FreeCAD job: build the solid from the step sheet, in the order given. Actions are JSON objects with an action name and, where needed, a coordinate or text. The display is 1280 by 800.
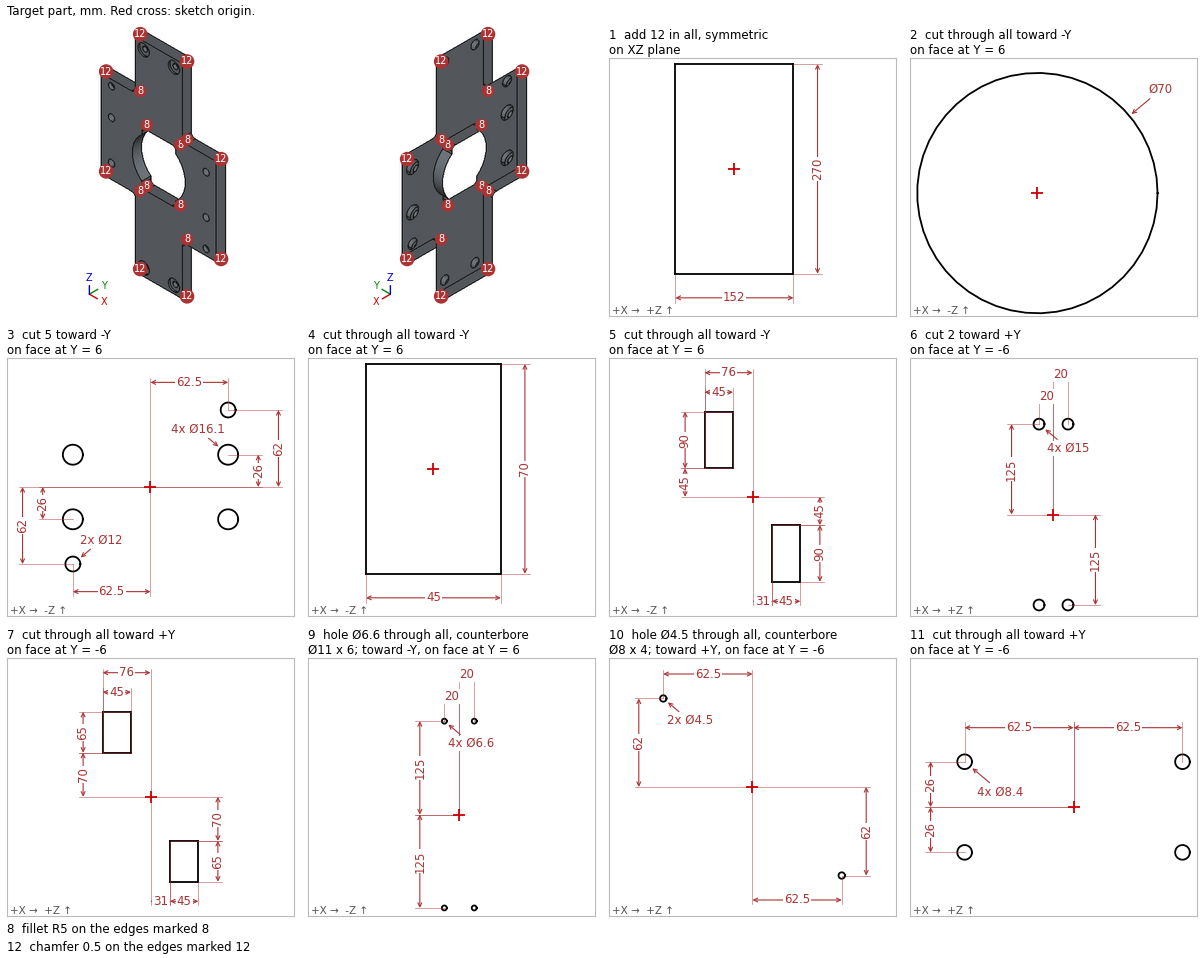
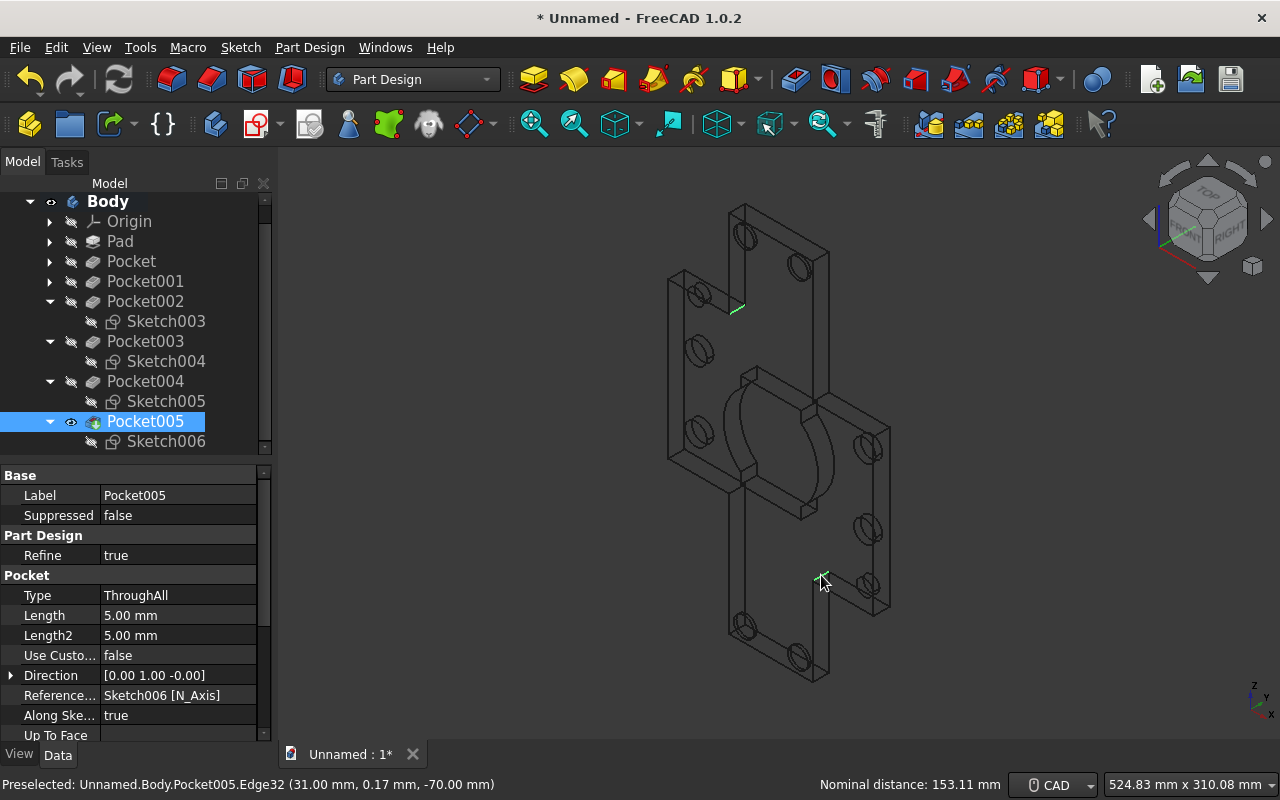
{"action": "left_click", "coordinate": [809, 514], "text": "ctrl"}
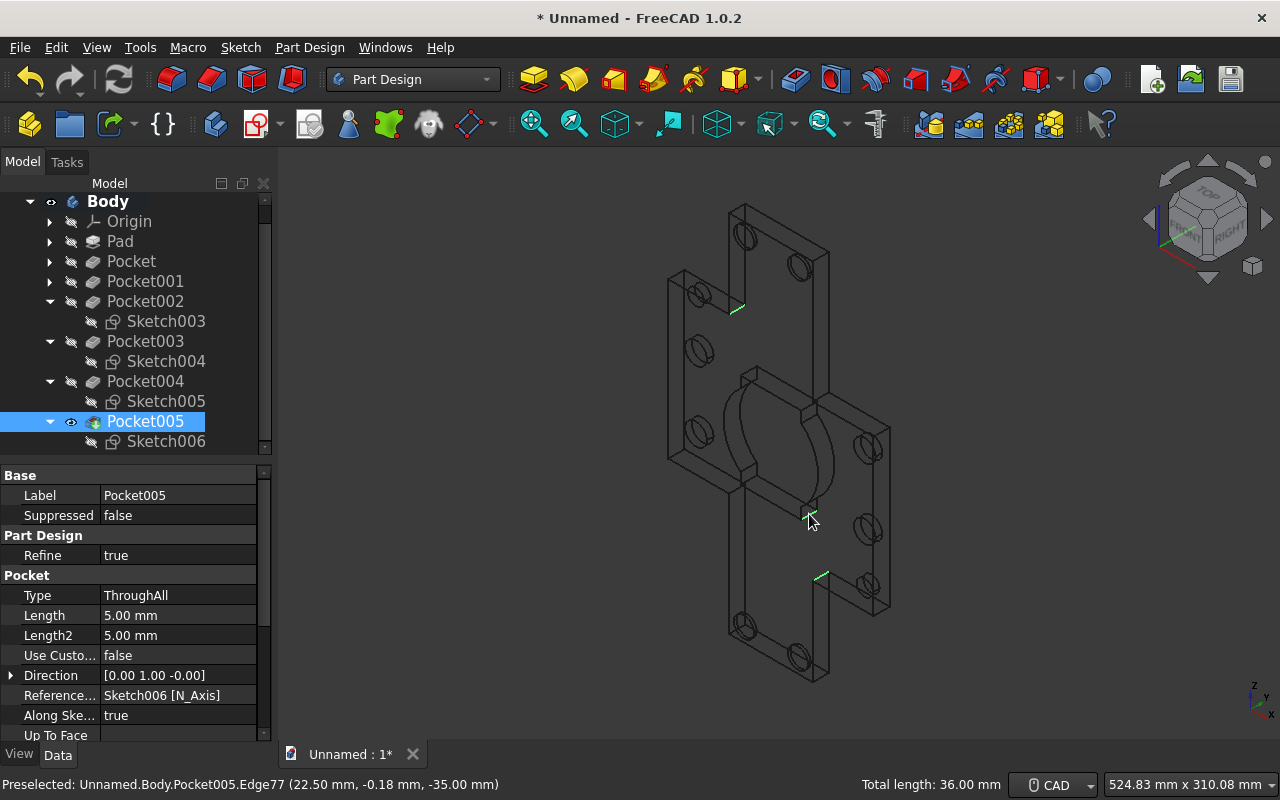
{"action": "left_click", "coordinate": [808, 406], "text": "ctrl"}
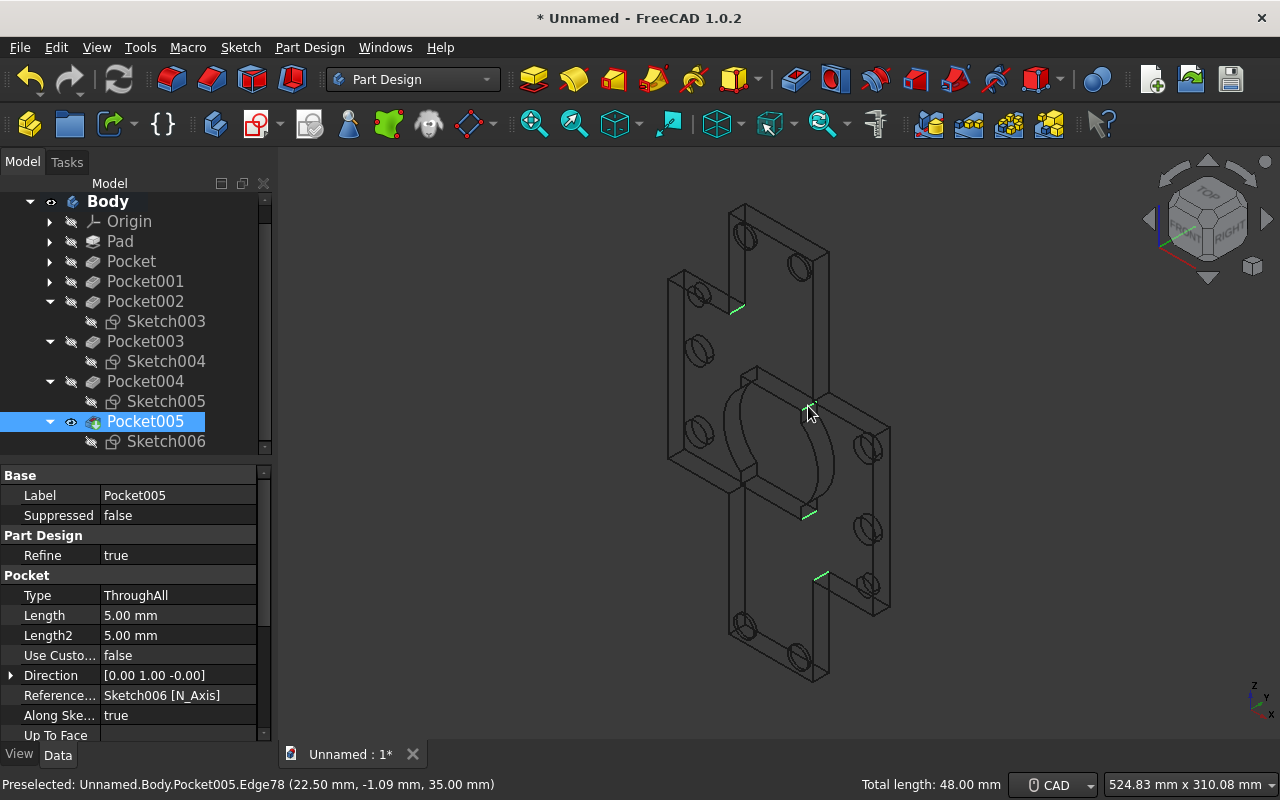
{"action": "left_click", "coordinate": [749, 370], "text": "ctrl"}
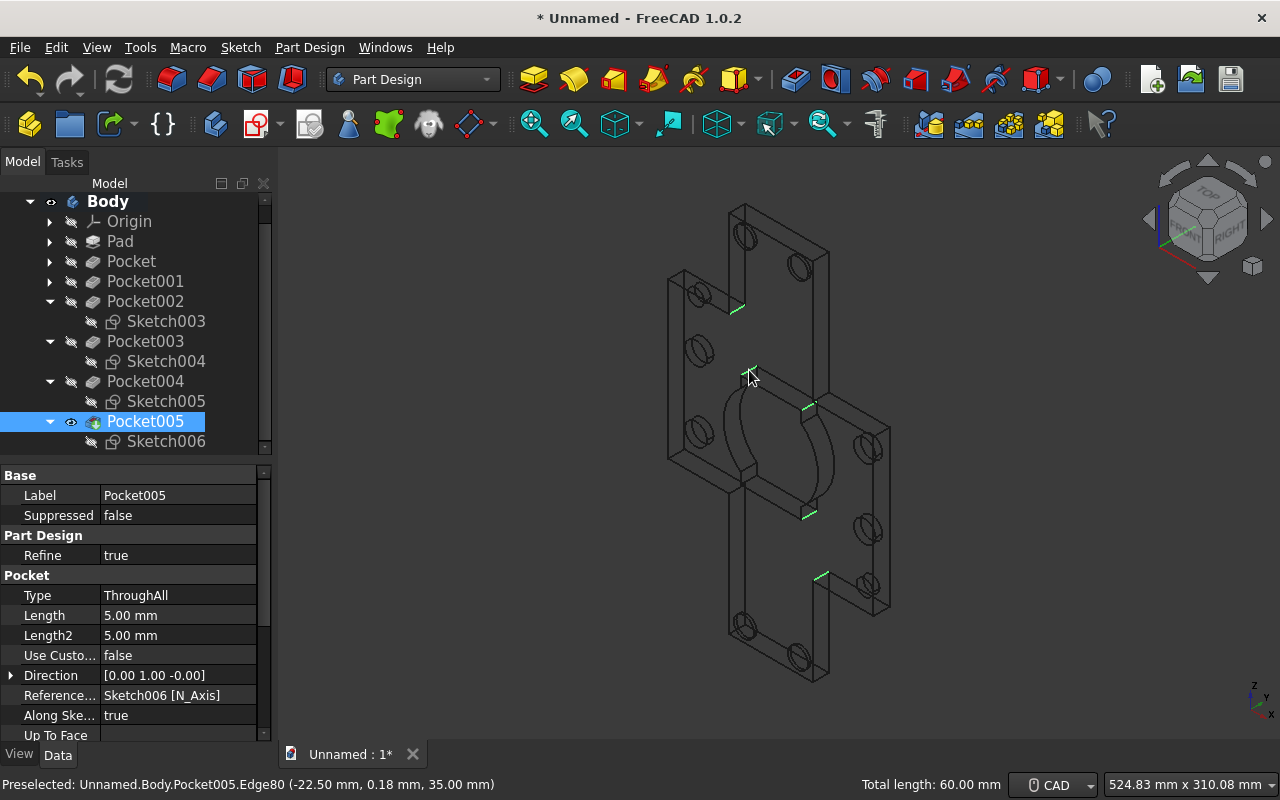
{"action": "left_click", "coordinate": [749, 479], "text": "ctrl"}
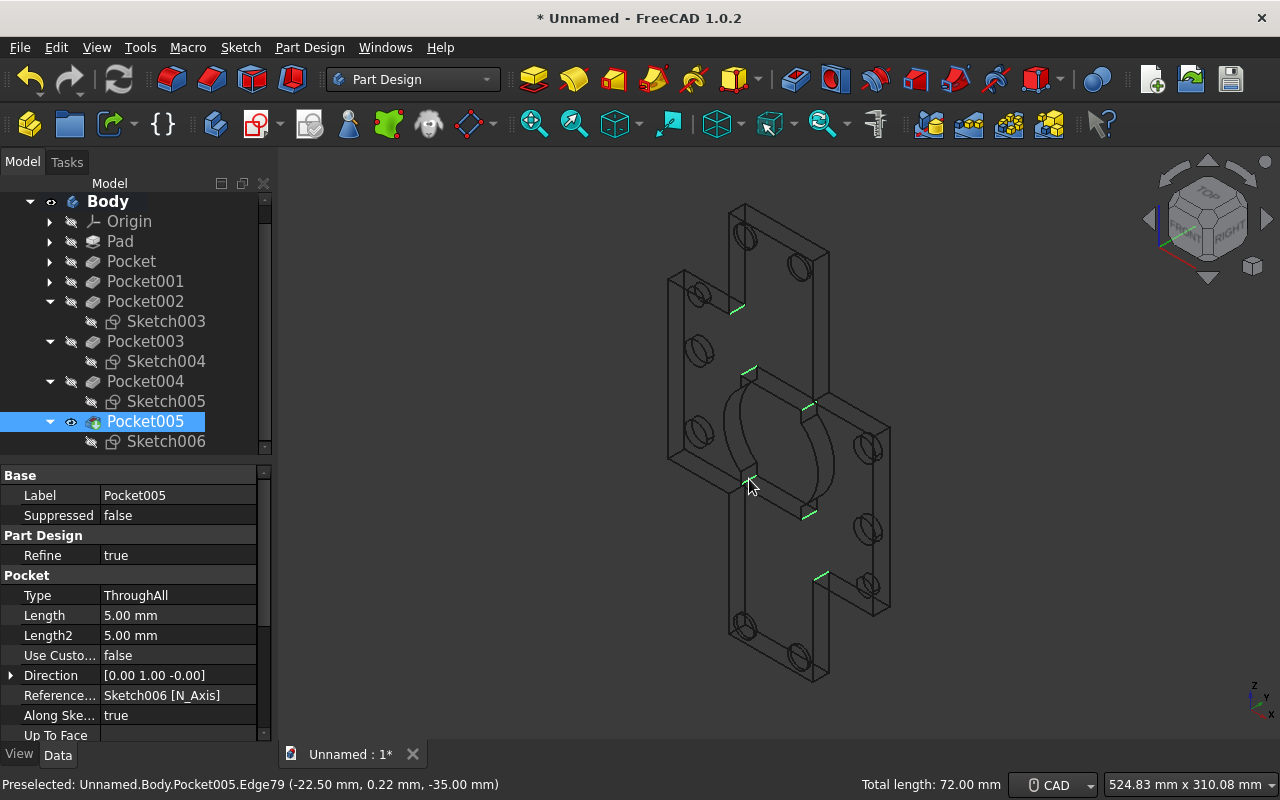
{"action": "left_click", "coordinate": [736, 489], "text": "ctrl"}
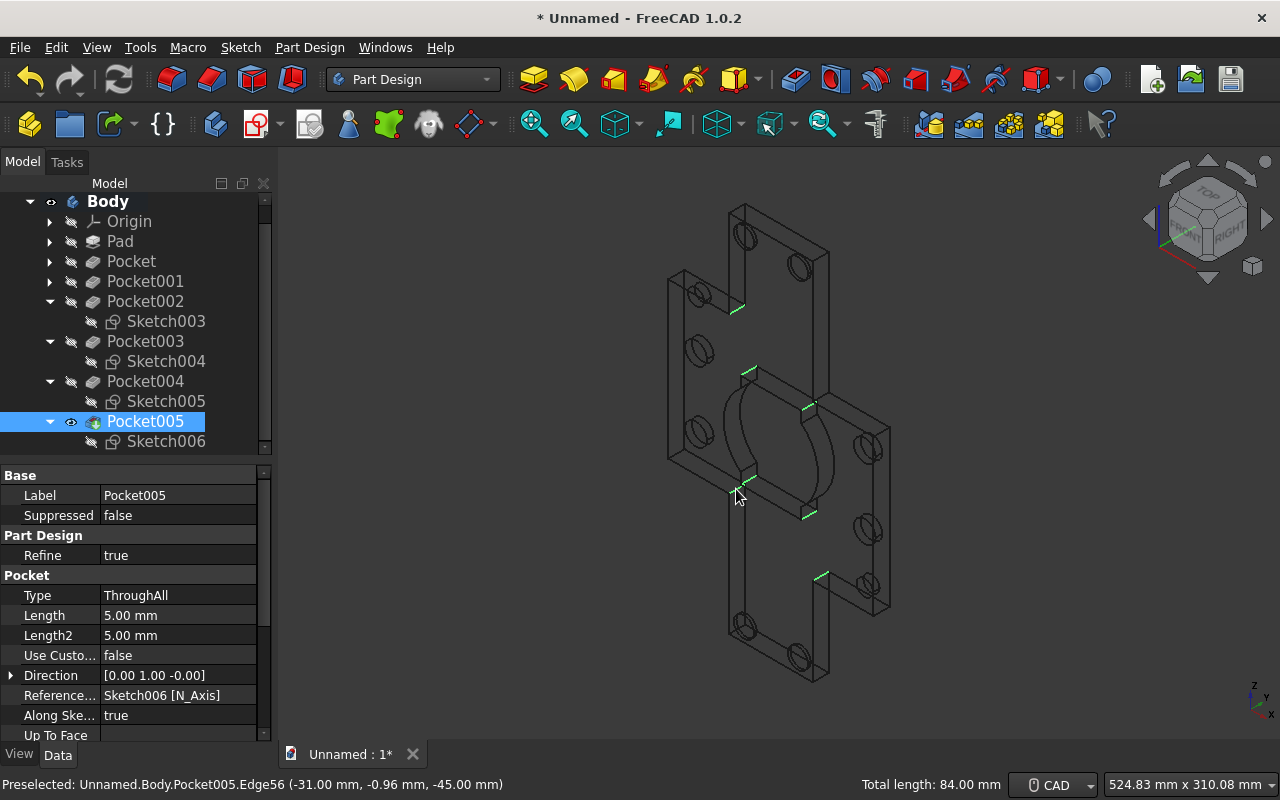
{"action": "left_click", "coordinate": [821, 396], "text": "ctrl"}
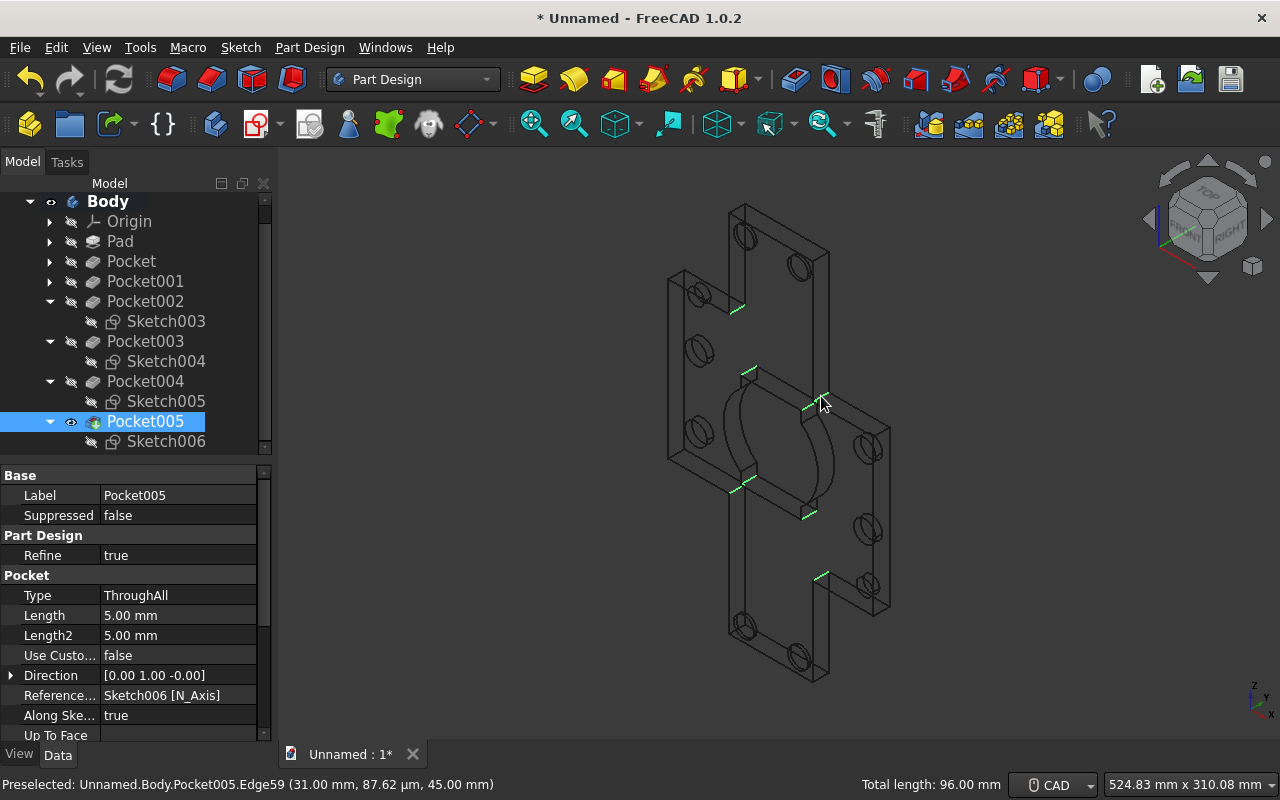
{"action": "key", "text": "v 1"}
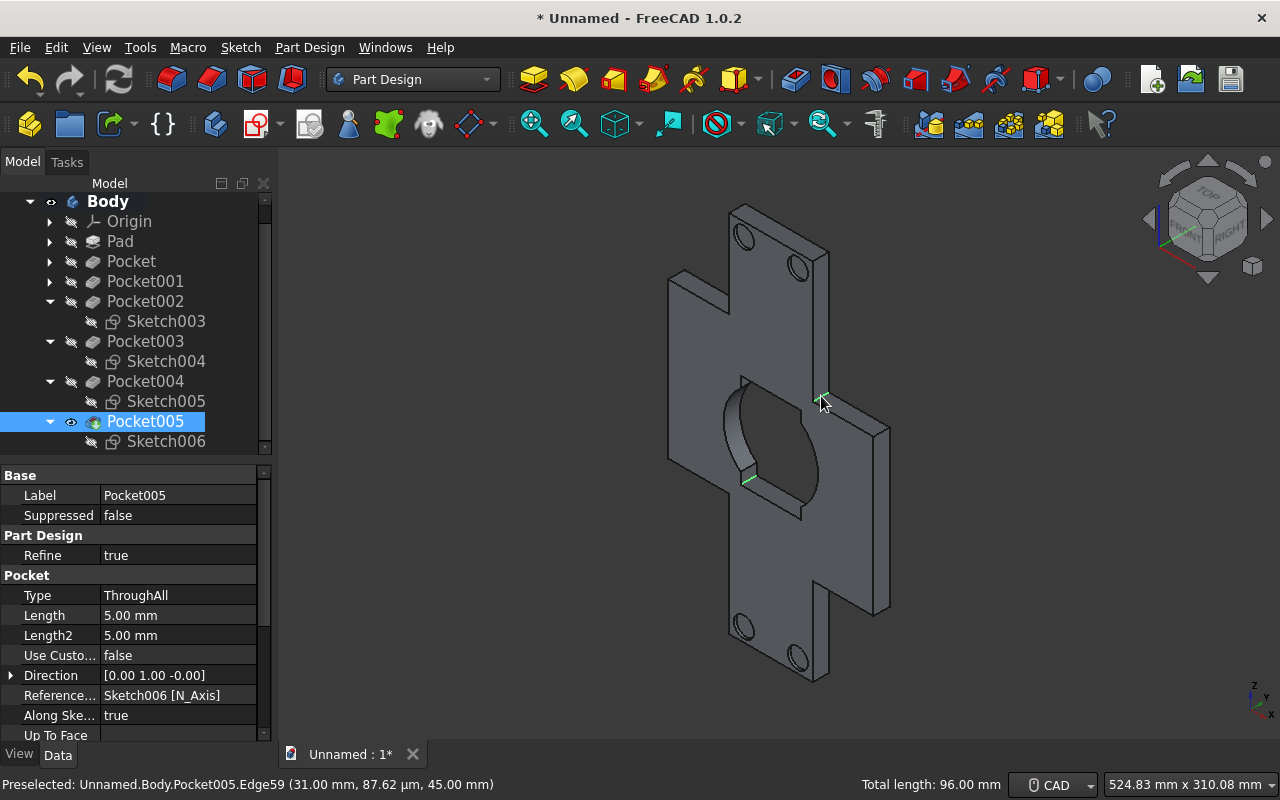
{"action": "left_click", "coordinate": [172, 80]}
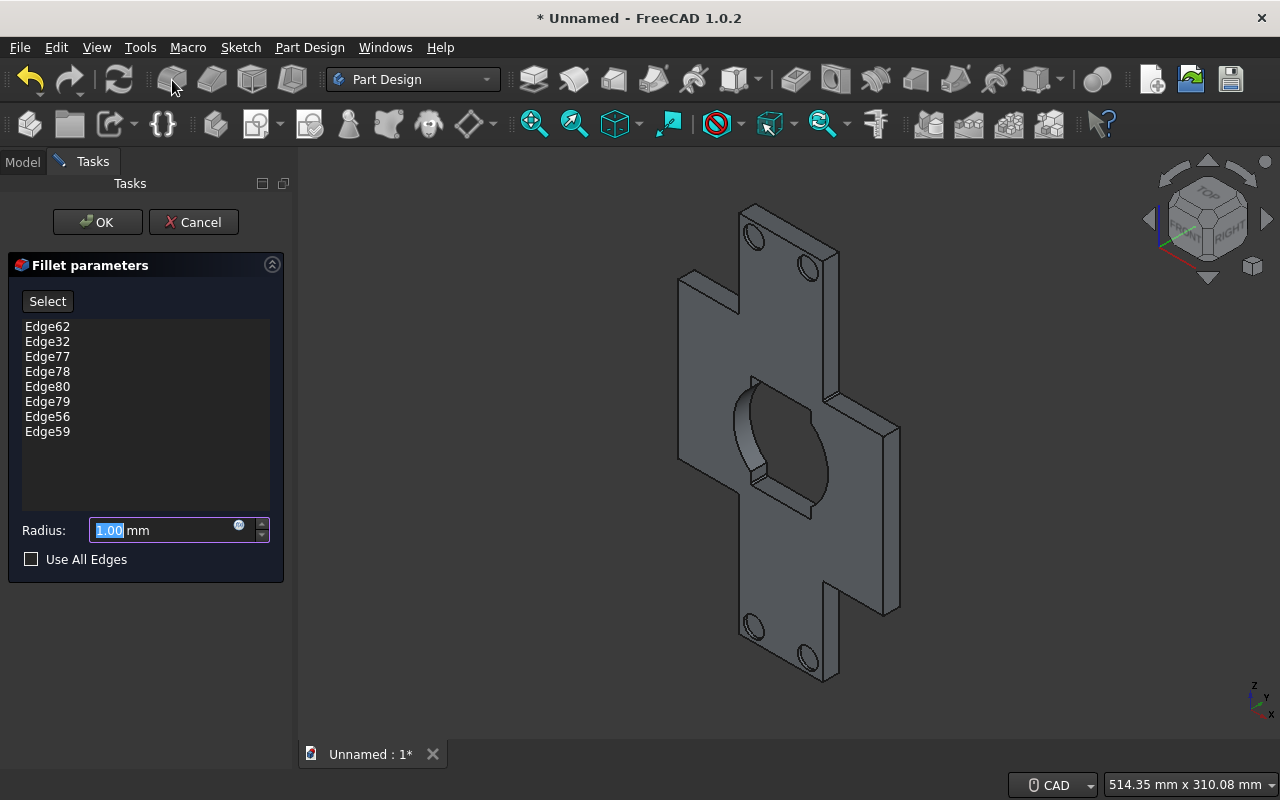
{"action": "type", "text": "5"}
{"action": "key", "text": "Tab"}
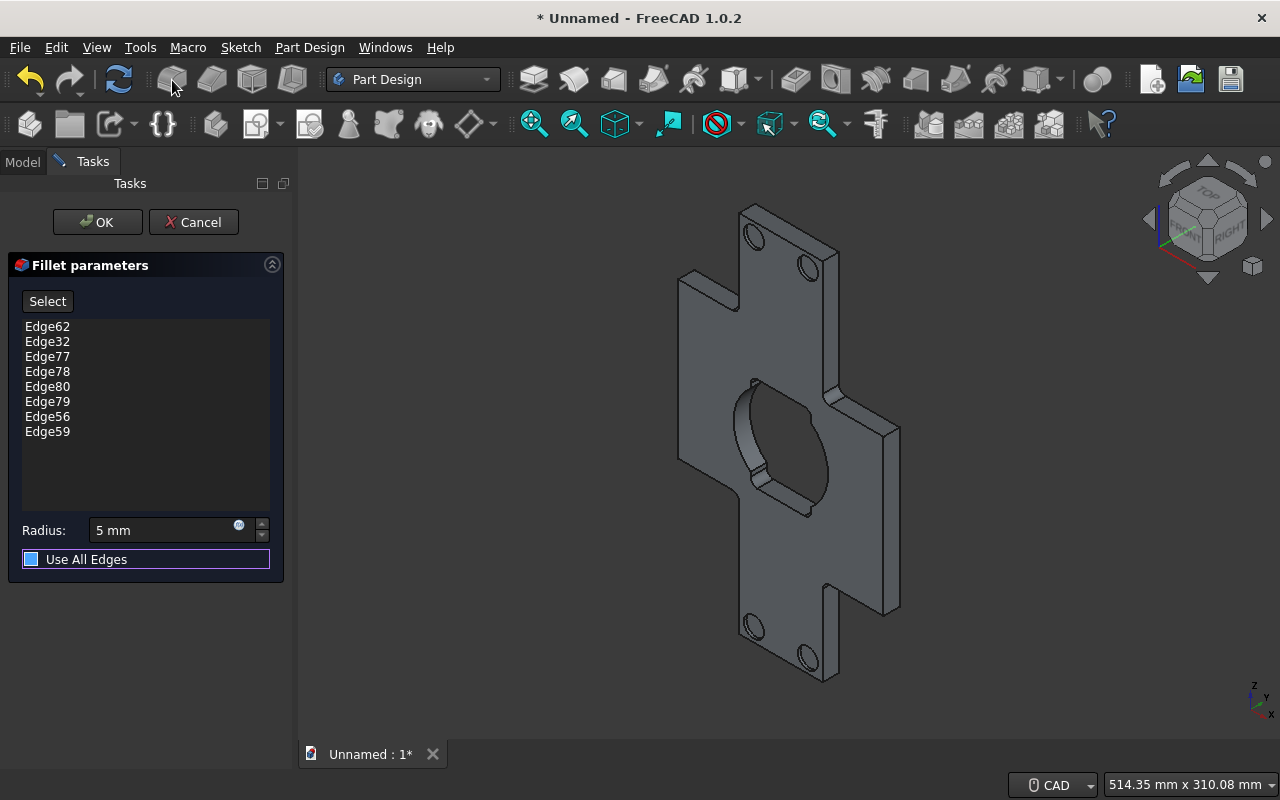
{"action": "left_click", "coordinate": [98, 222]}